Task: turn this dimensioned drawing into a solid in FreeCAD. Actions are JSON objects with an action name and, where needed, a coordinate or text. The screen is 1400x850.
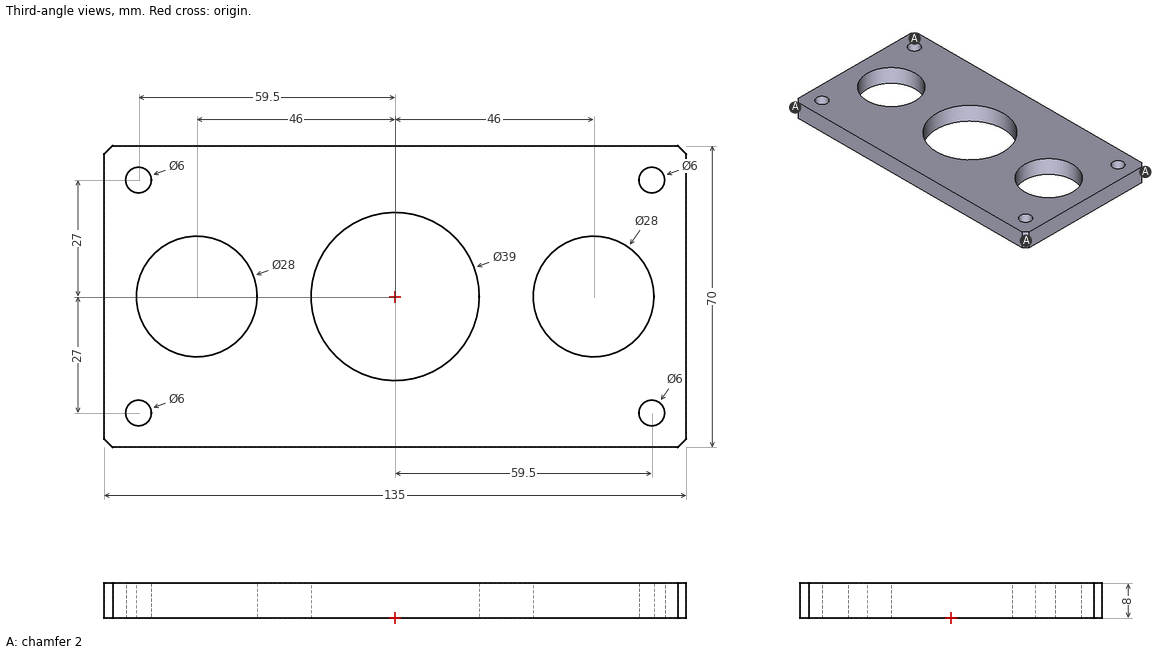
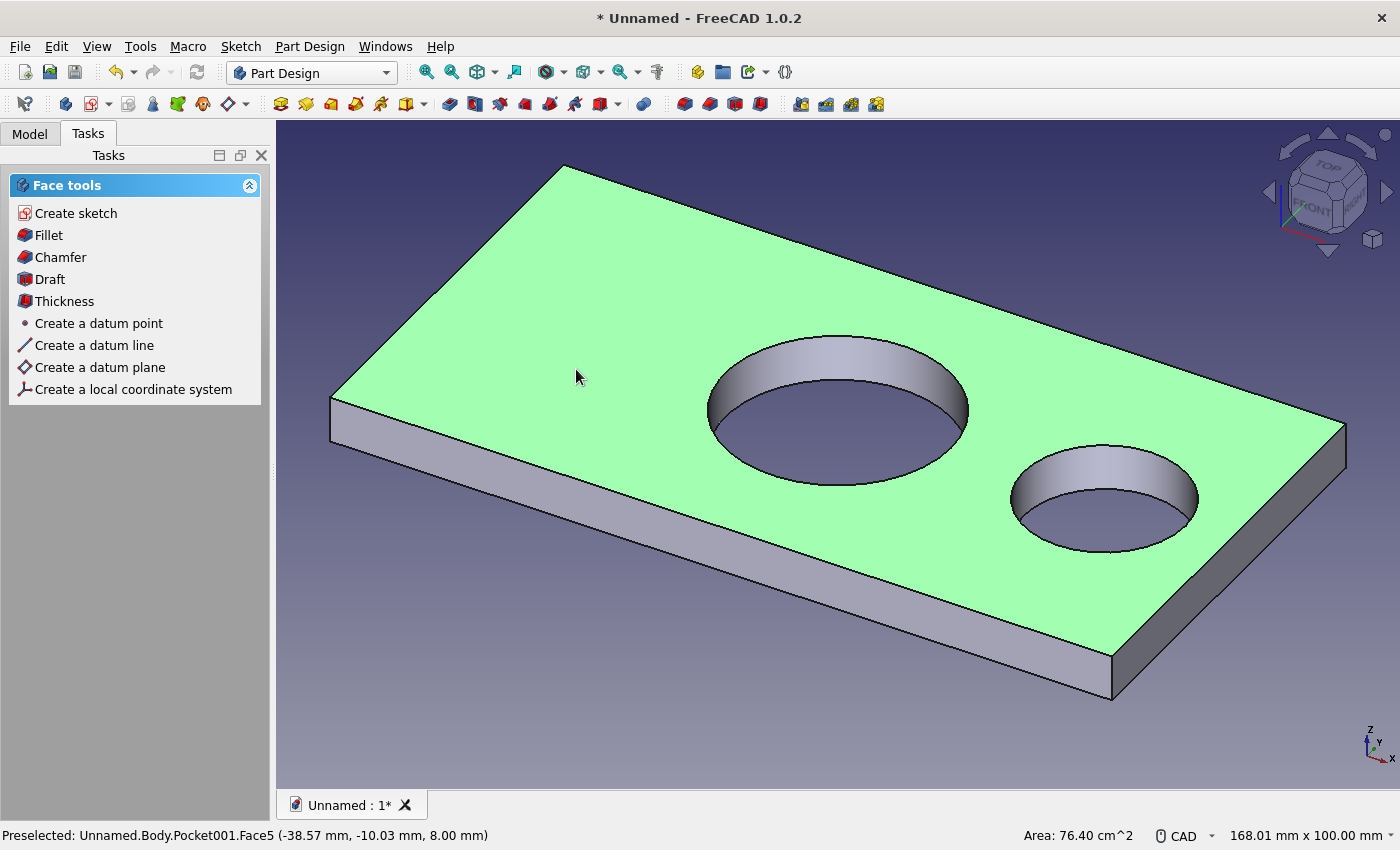
{"action": "left_click", "coordinate": [90, 104]}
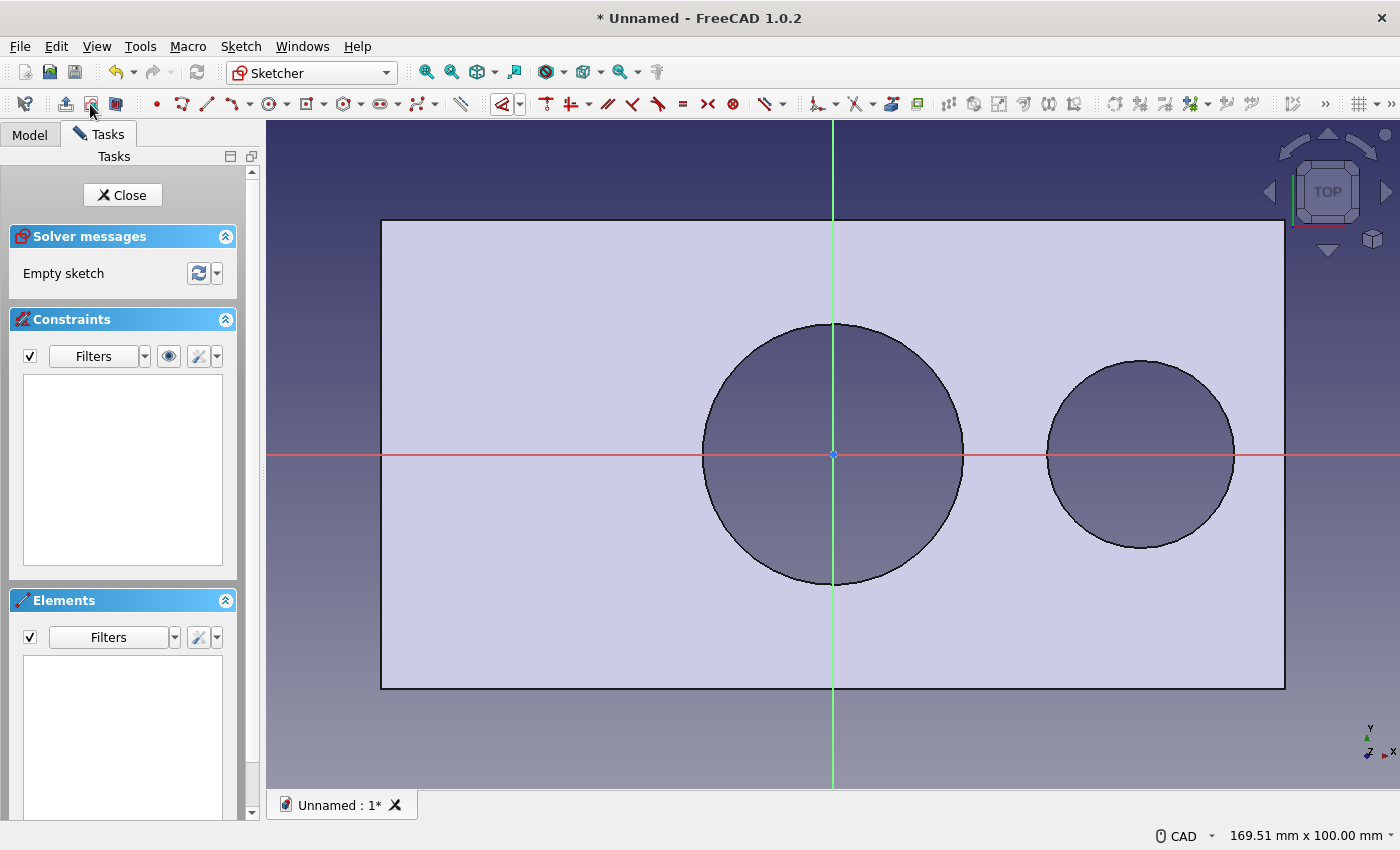
{"action": "scroll", "coordinate": [471, 454], "scroll_direction": "up", "scroll_amount": 3}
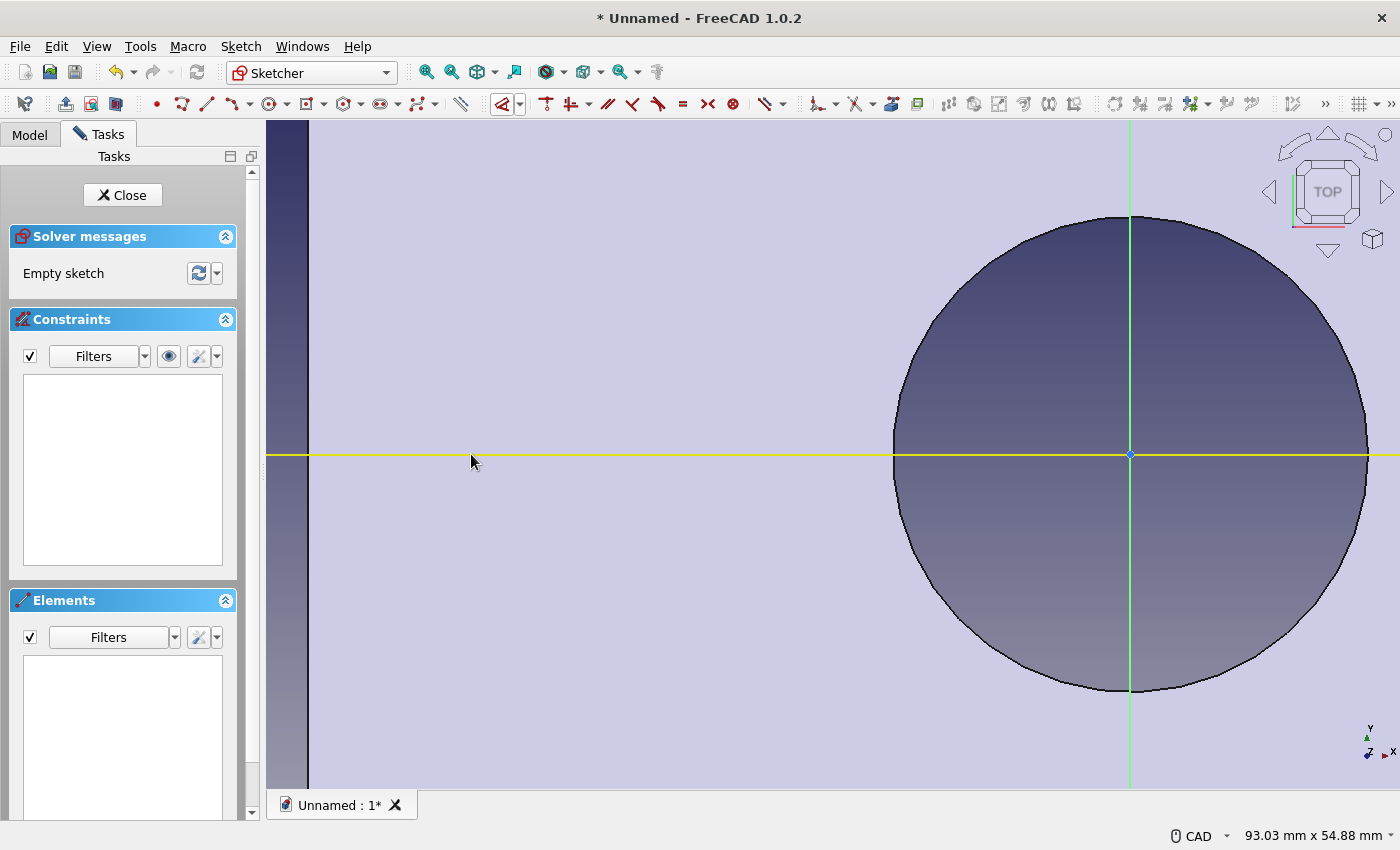
{"action": "key", "text": "g c"}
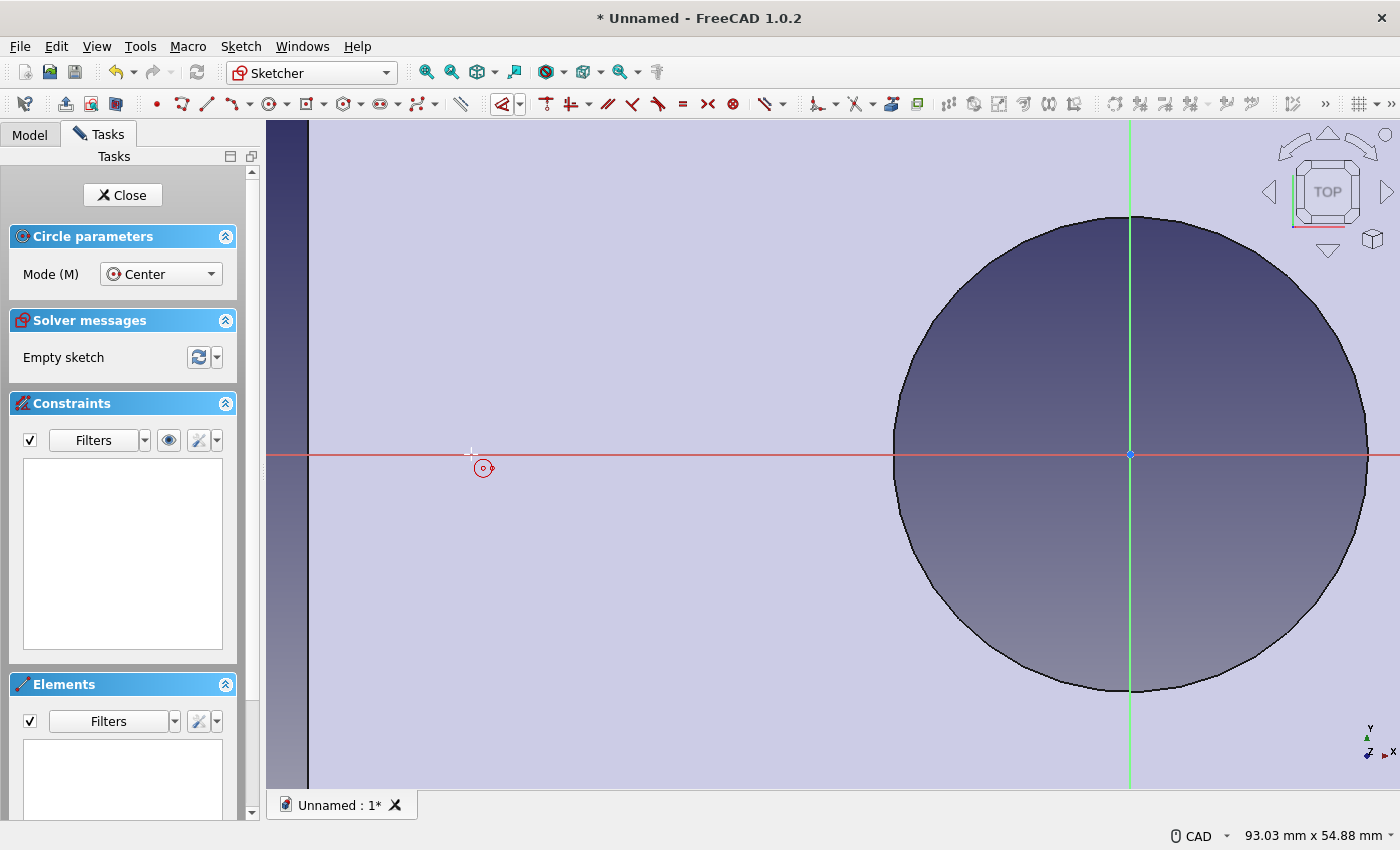
{"action": "left_click", "coordinate": [570, 454]}
{"action": "left_click", "coordinate": [690, 334]}
{"action": "key", "text": "Escape"}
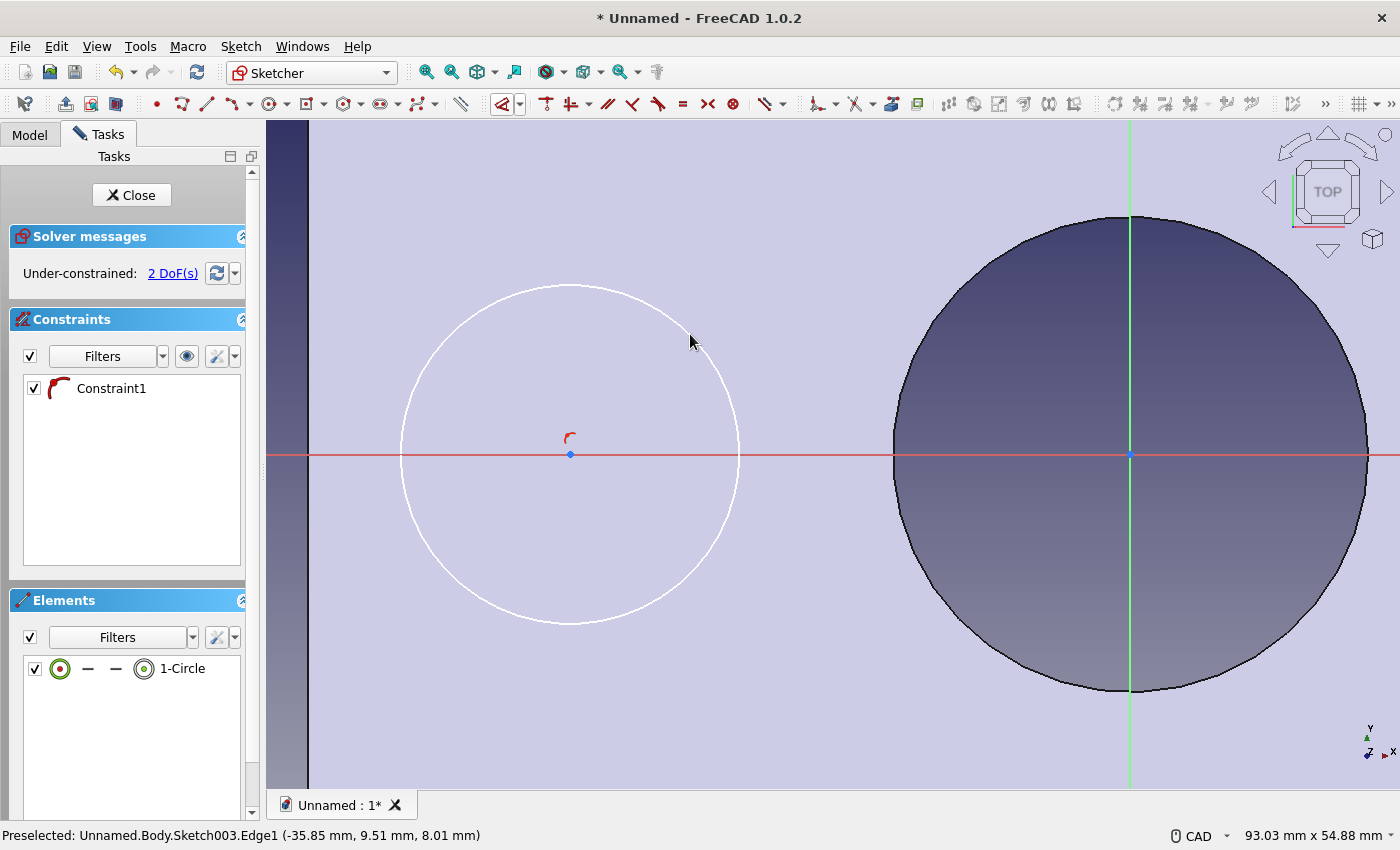
{"action": "left_click", "coordinate": [689, 334]}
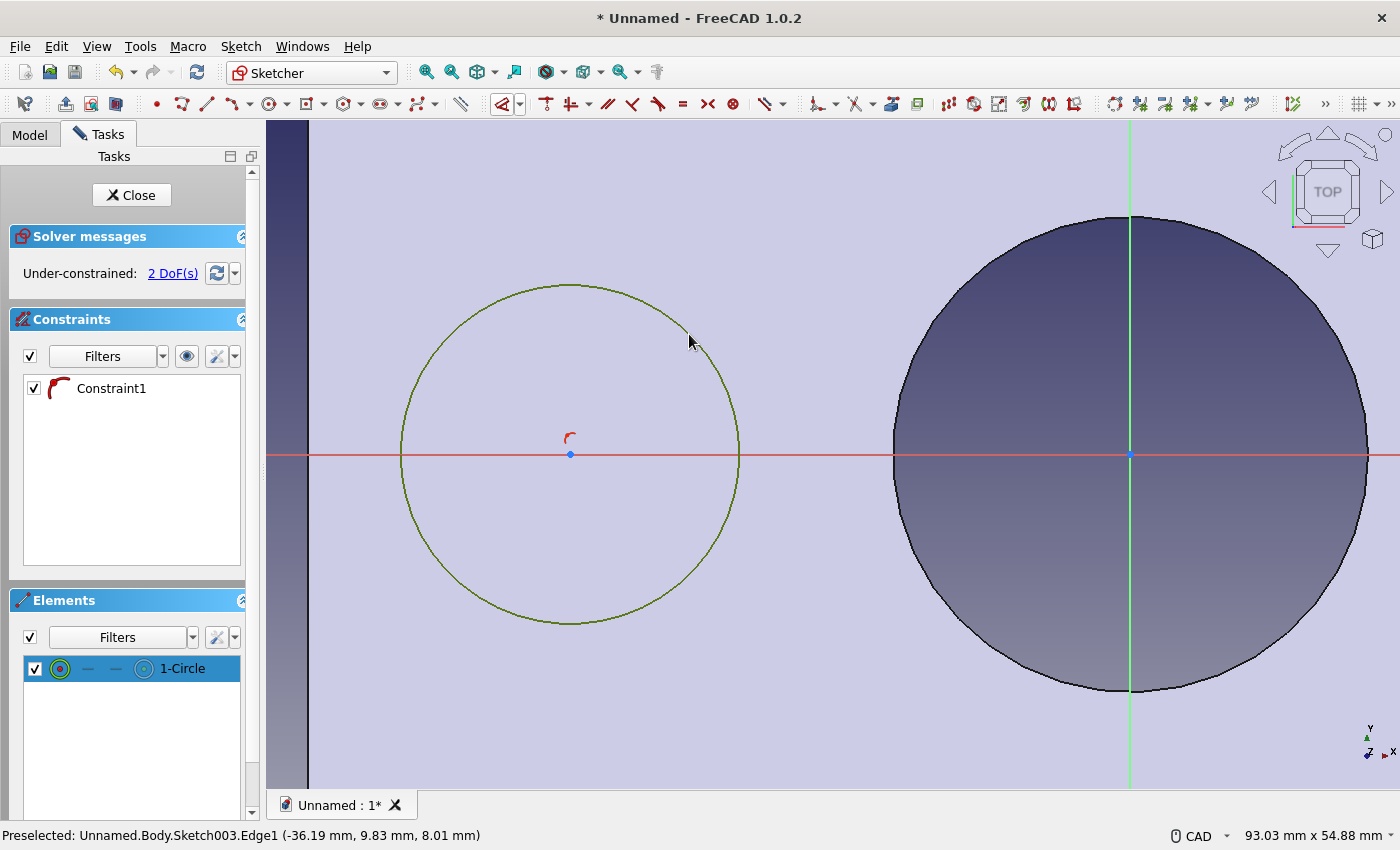
{"action": "key", "text": "k o"}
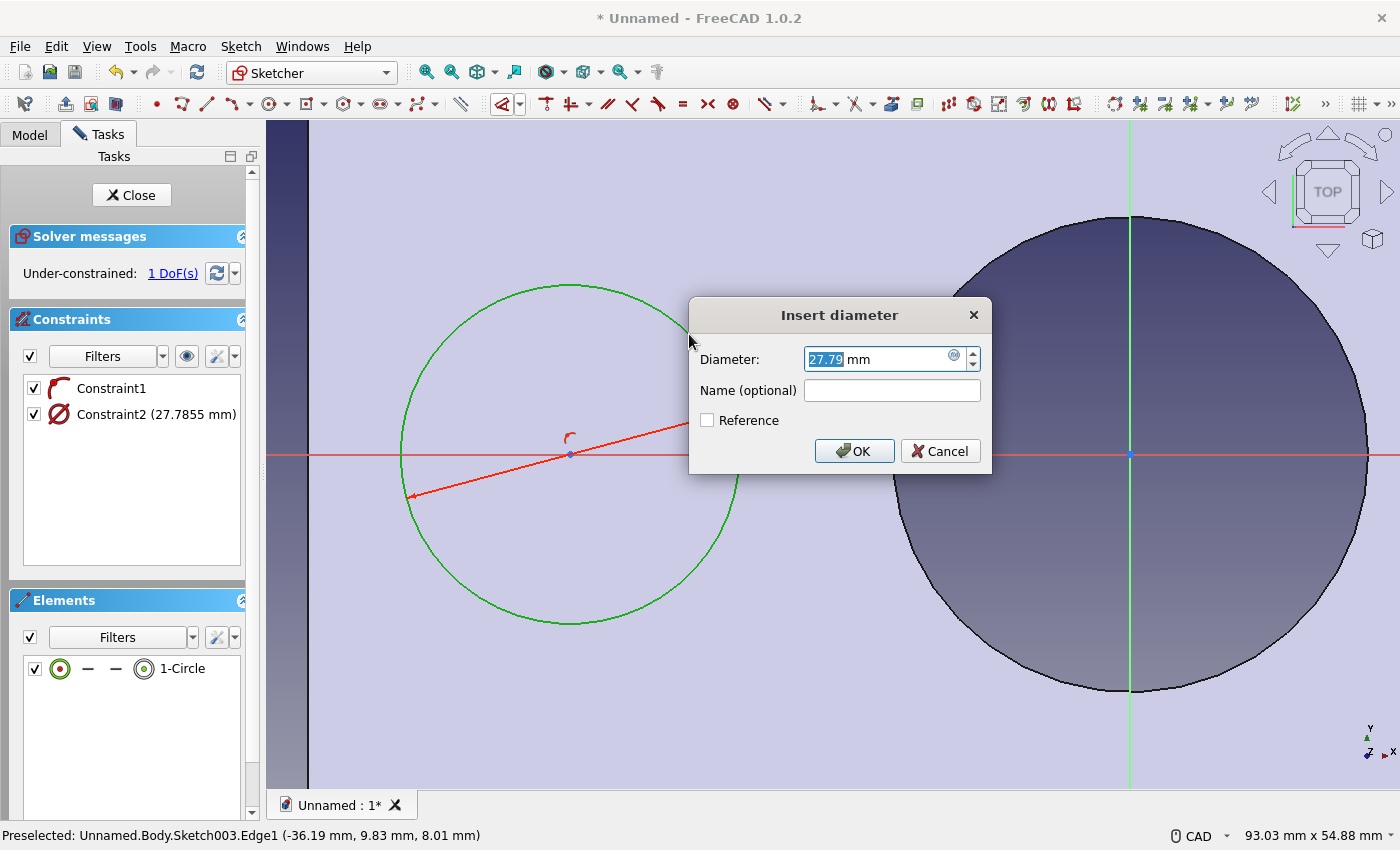
{"action": "type", "text": "28"}
{"action": "key", "text": "Return"}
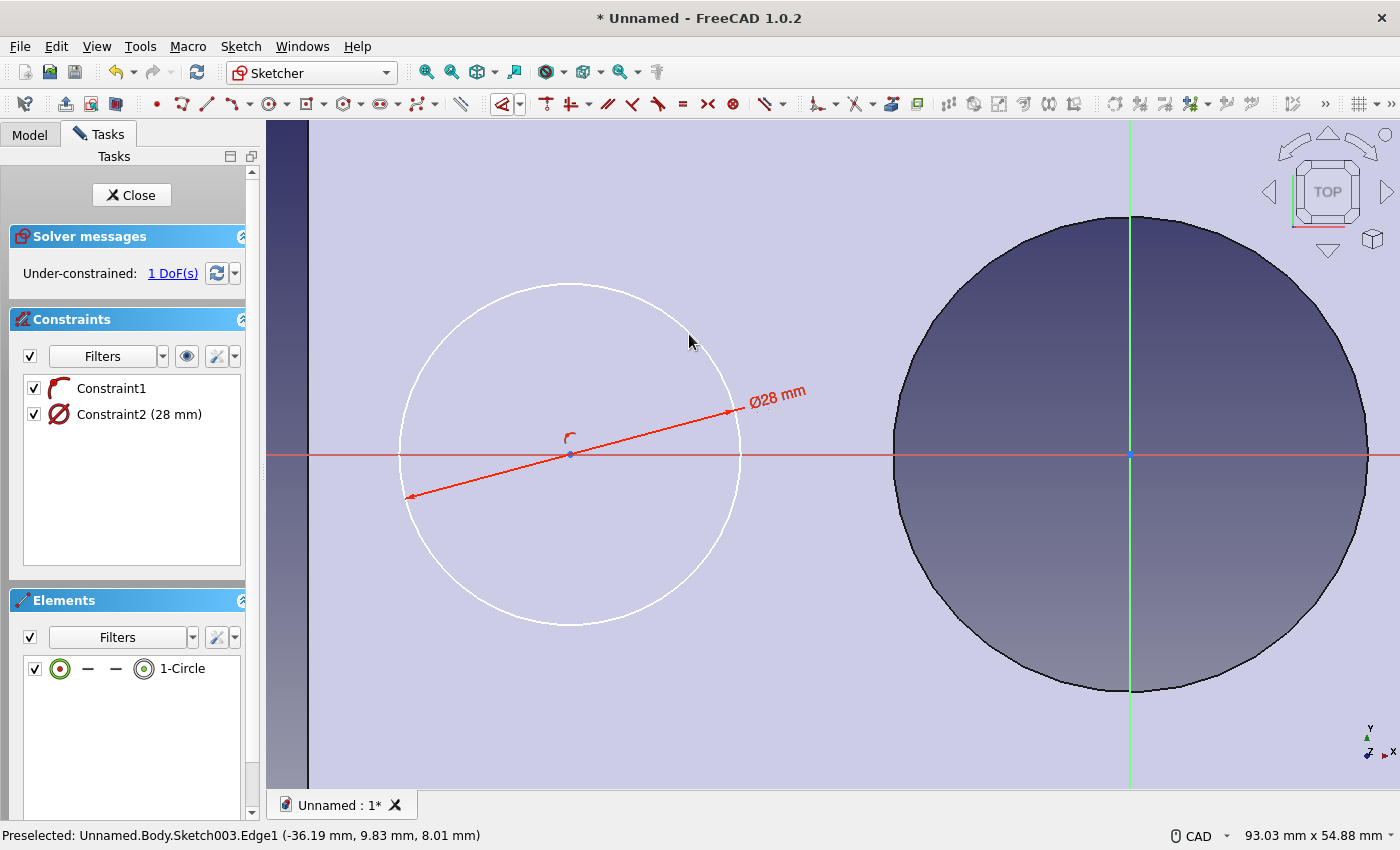
{"action": "left_click", "coordinate": [570, 454]}